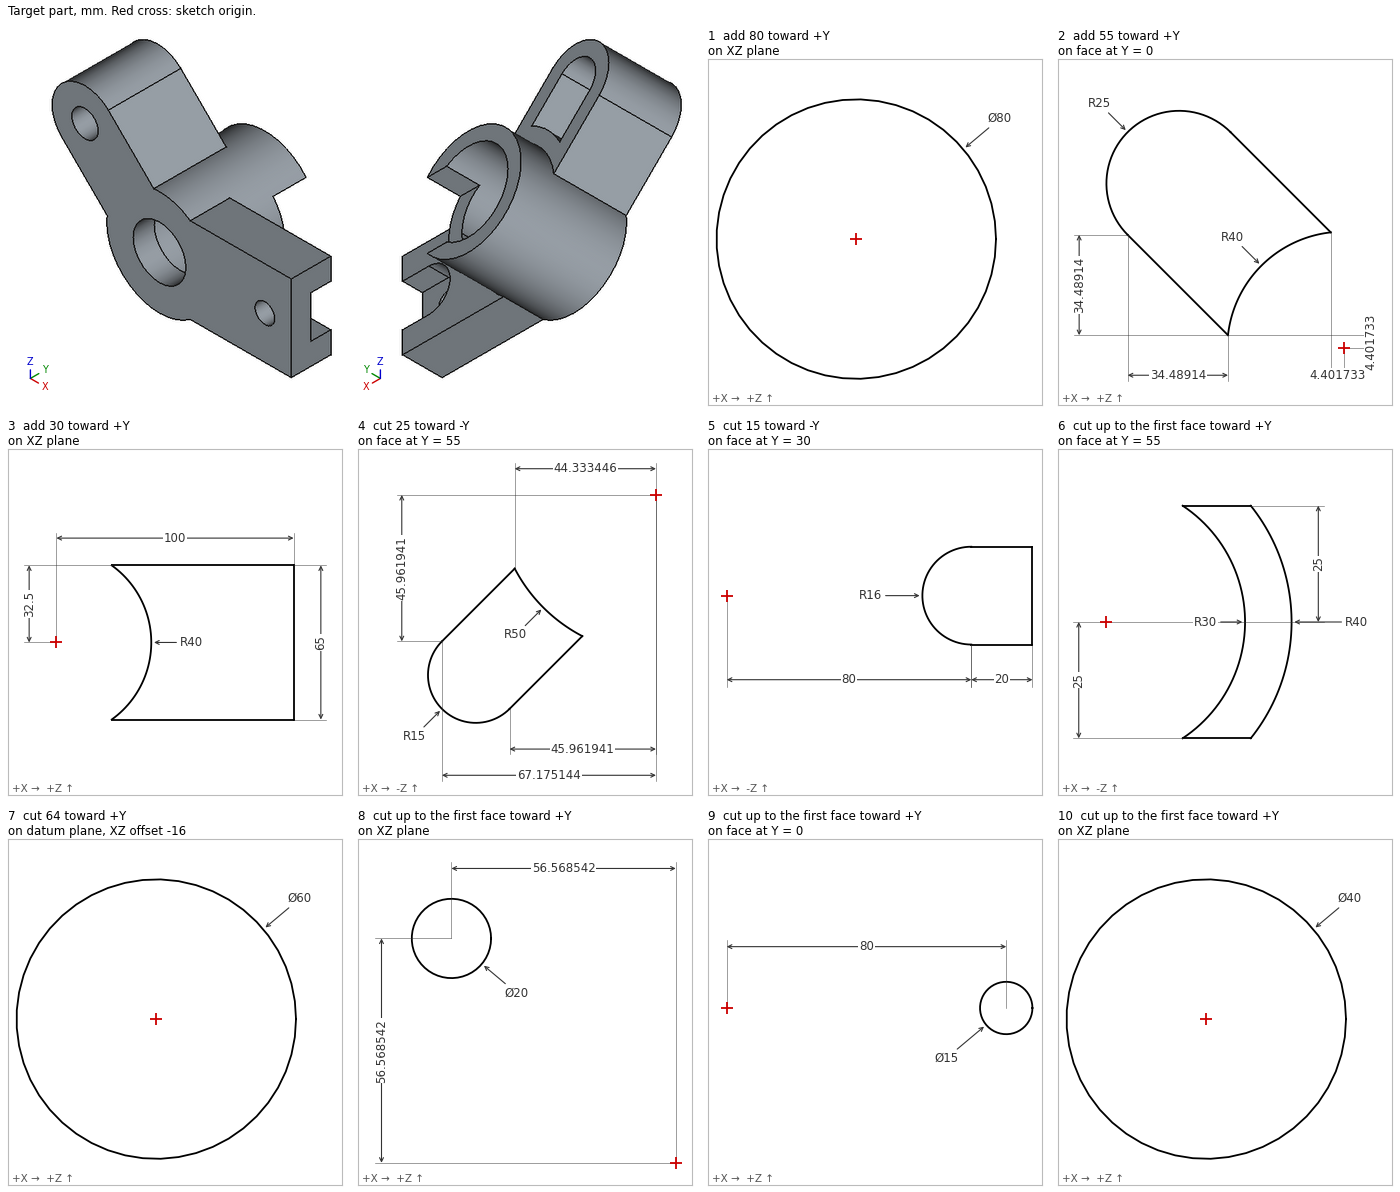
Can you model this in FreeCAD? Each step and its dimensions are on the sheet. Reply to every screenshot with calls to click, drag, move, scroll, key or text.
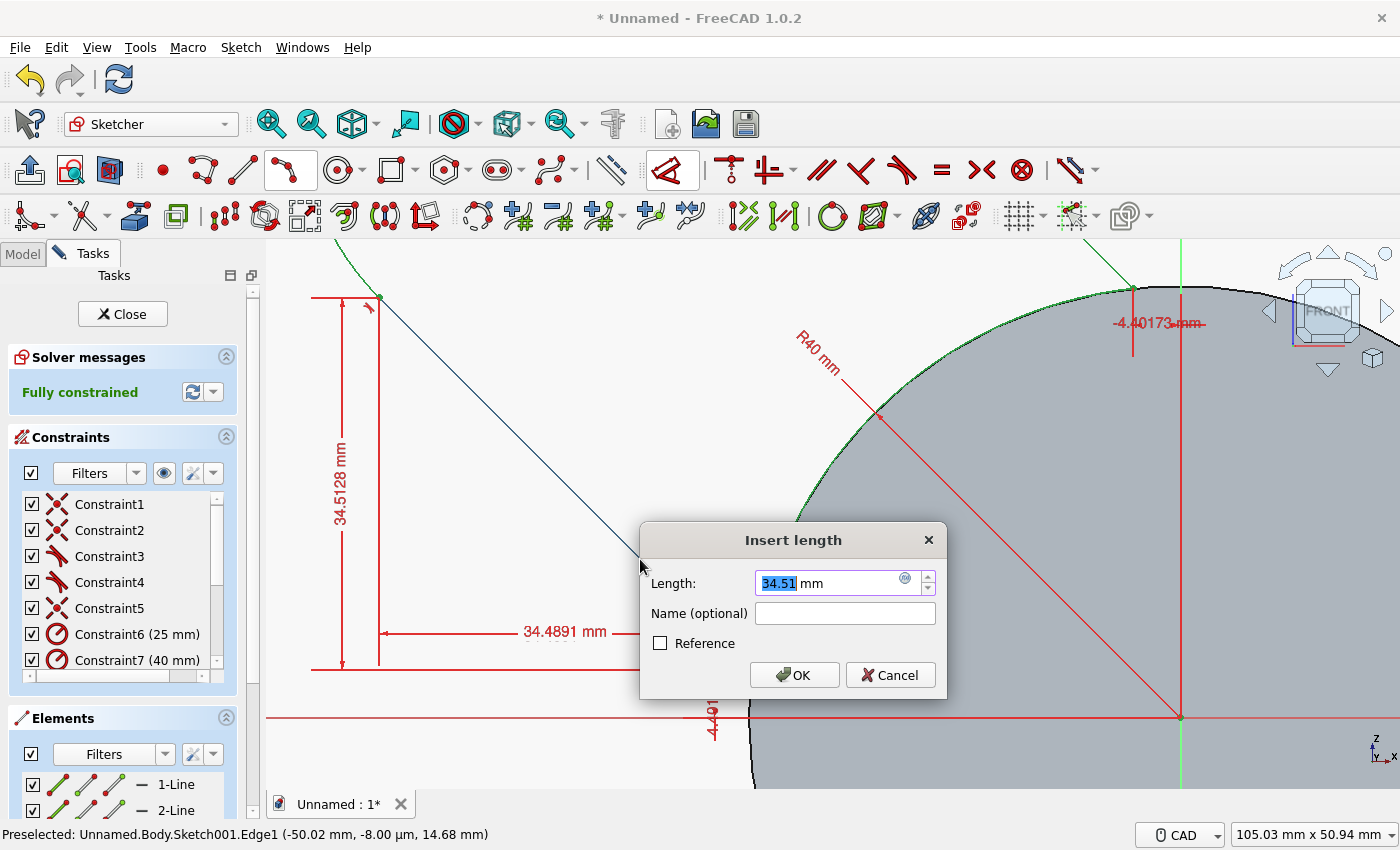
text(34.48914)
key(Return)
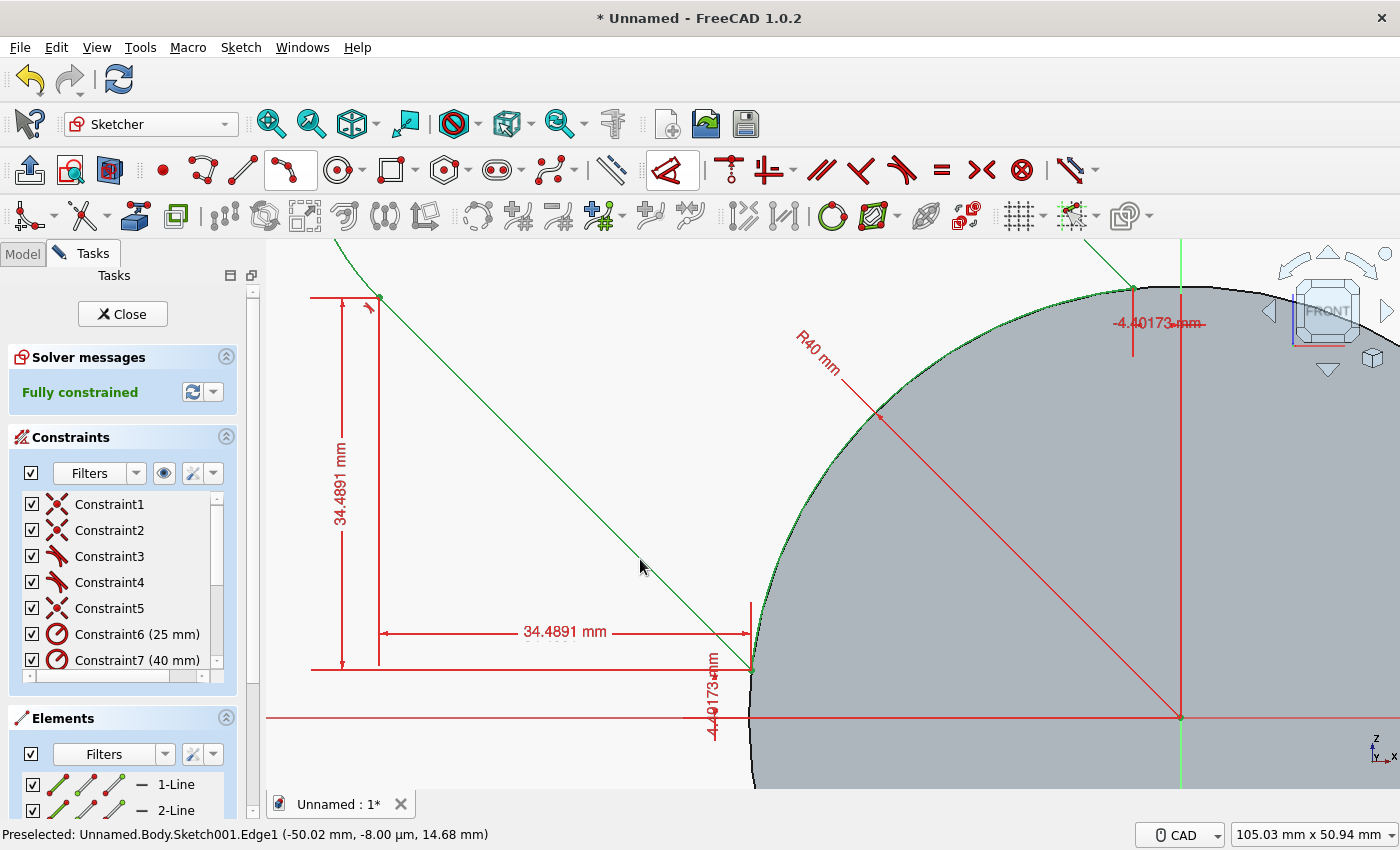
click(123, 314)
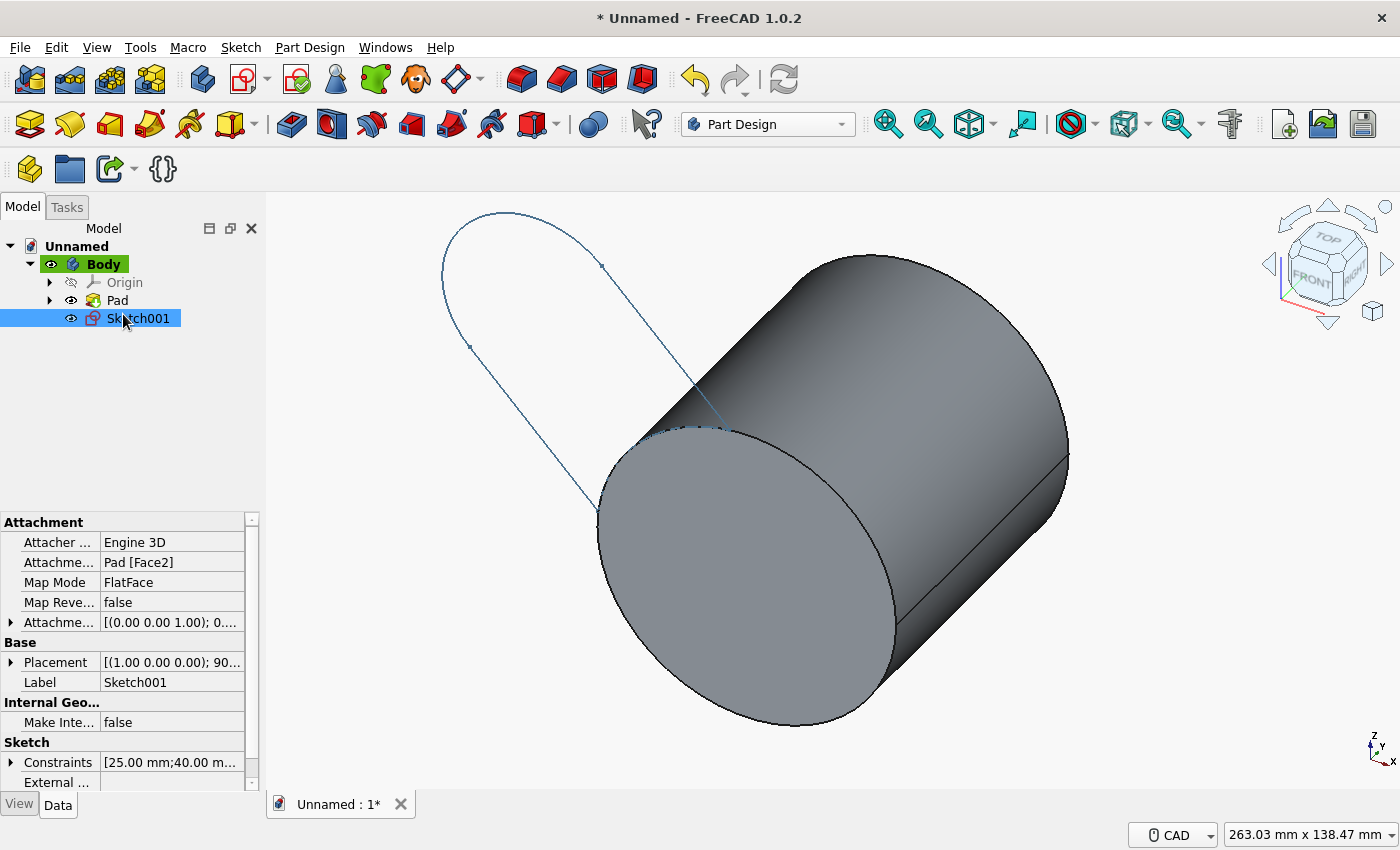
click(30, 124)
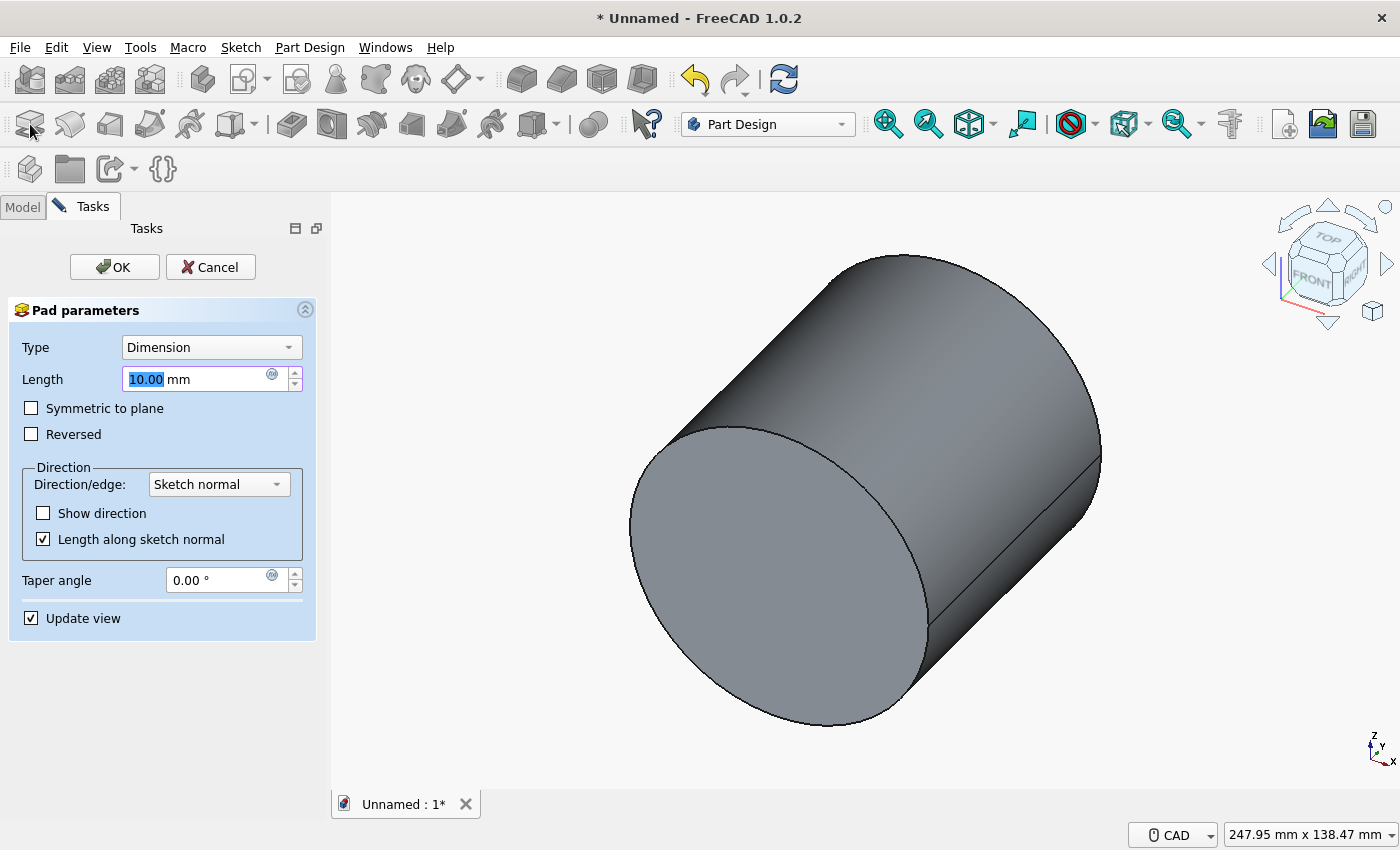
text(55)
key(Tab)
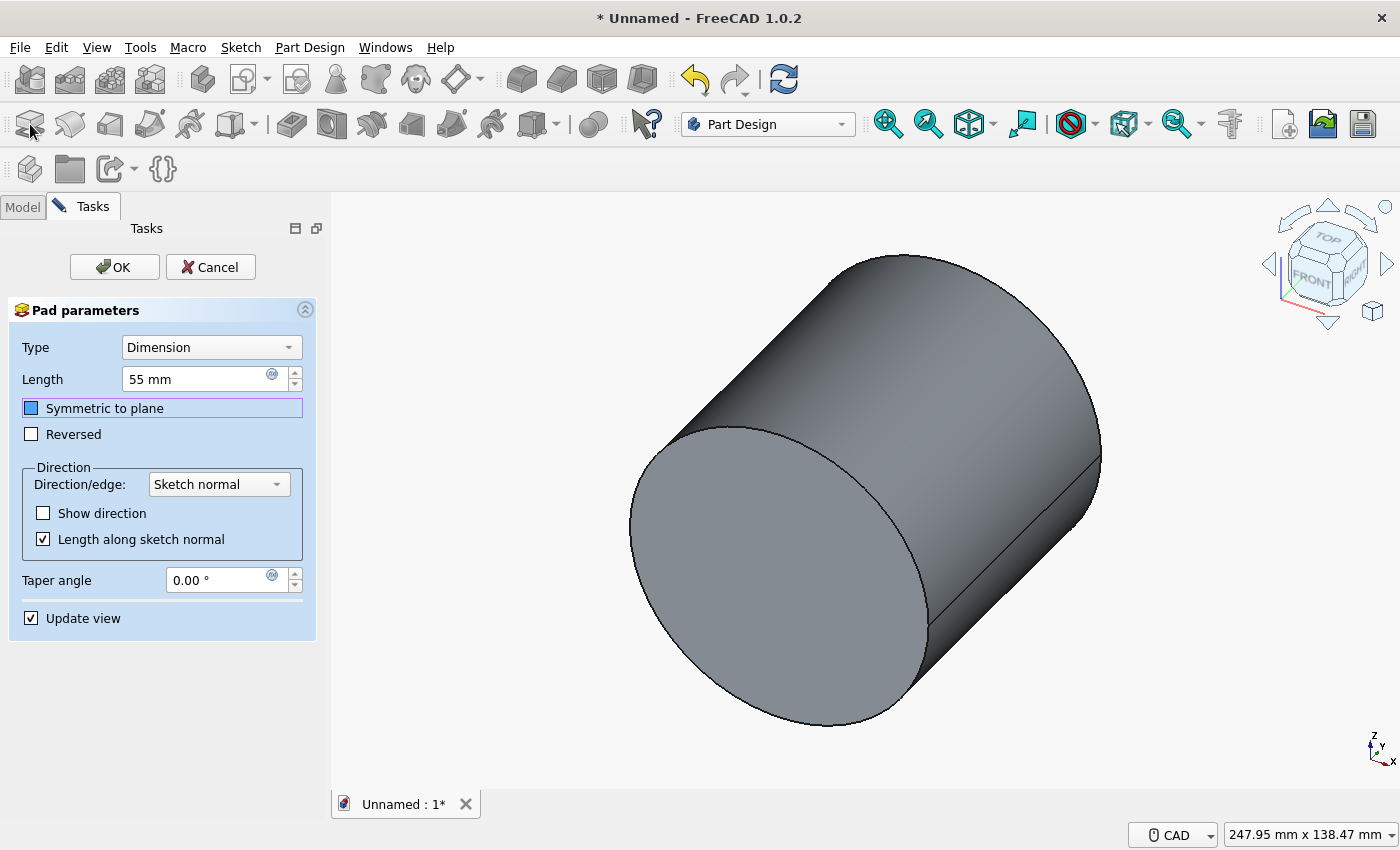
click(30, 434)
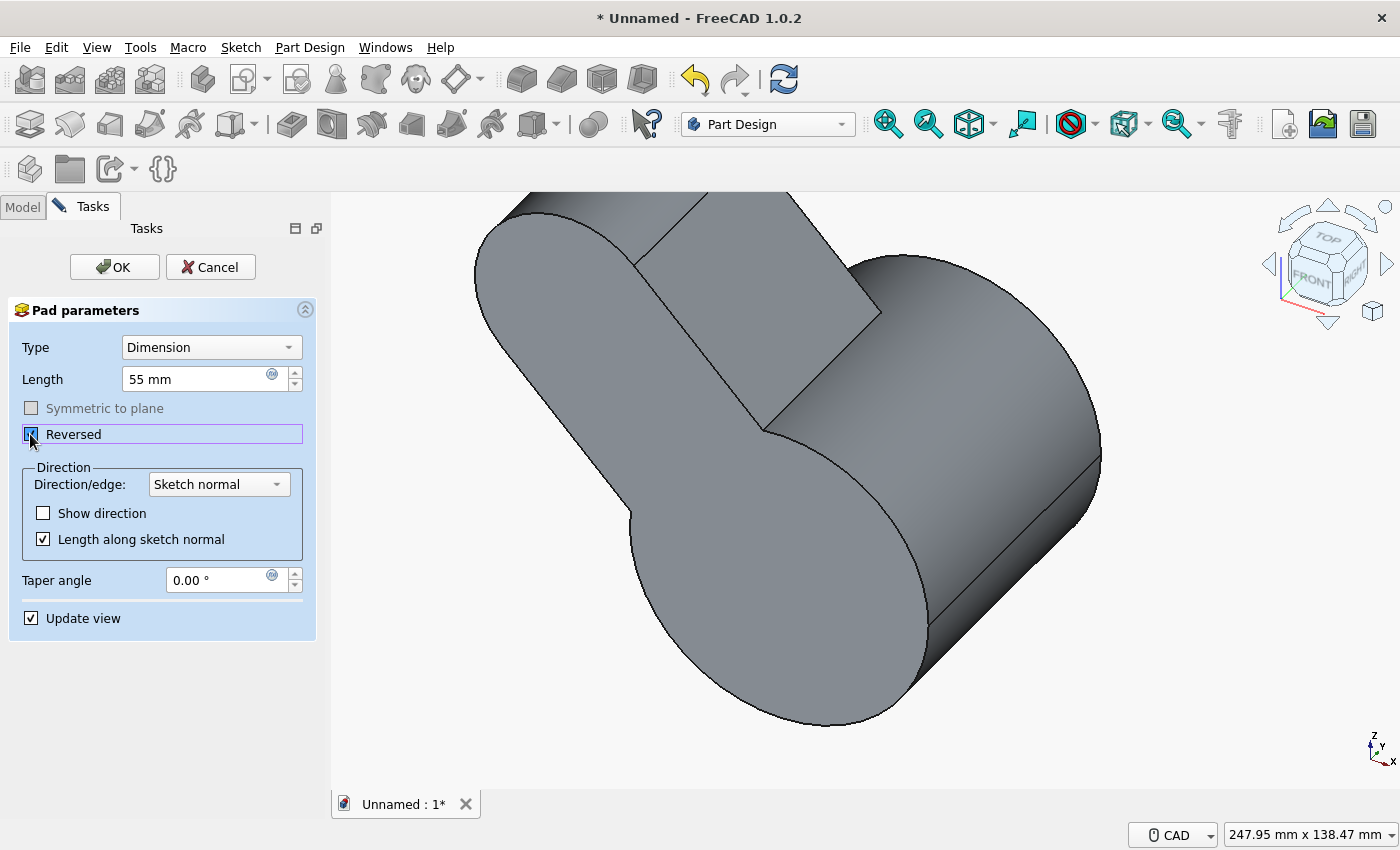
click(115, 267)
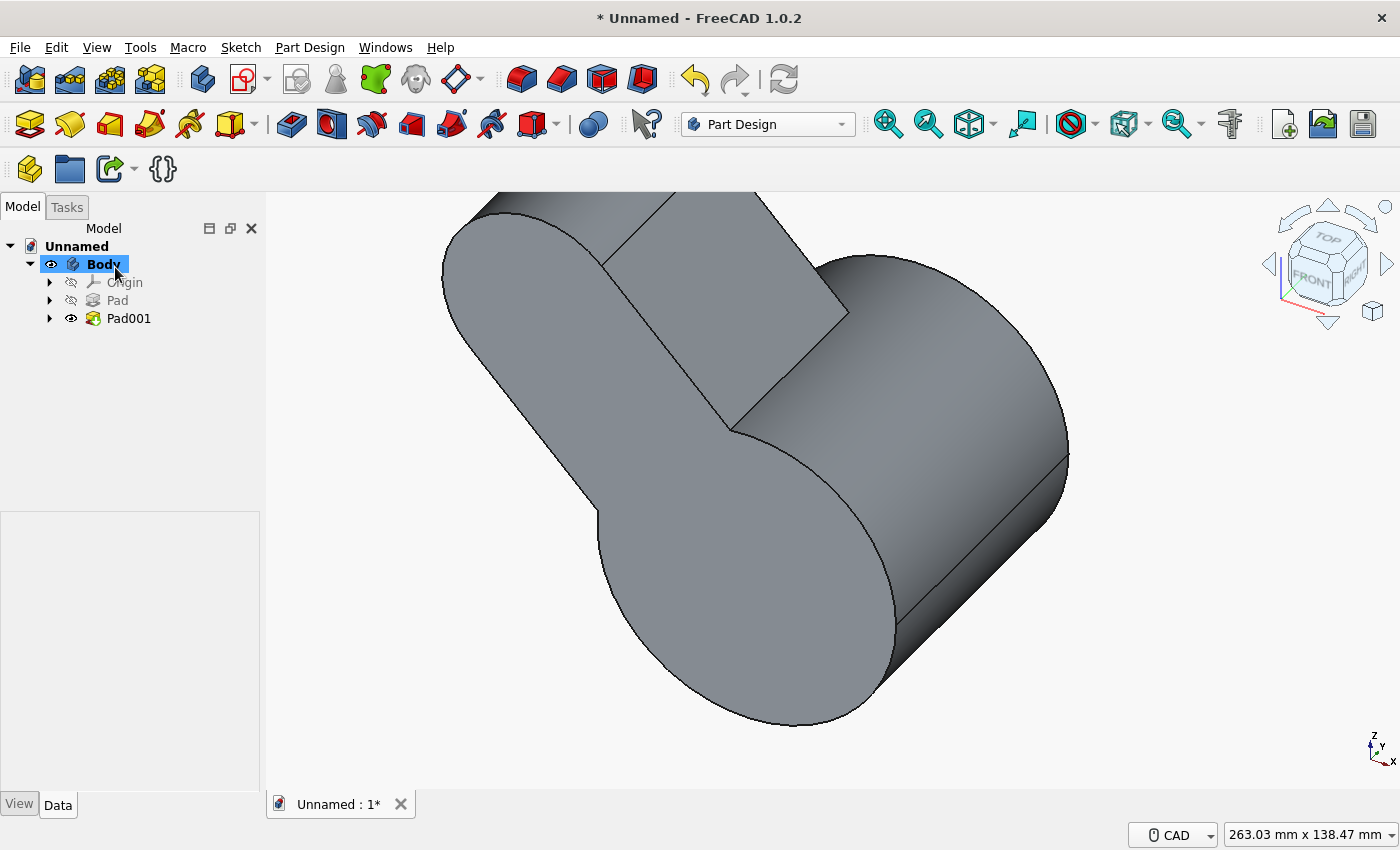
key(v)
key(f)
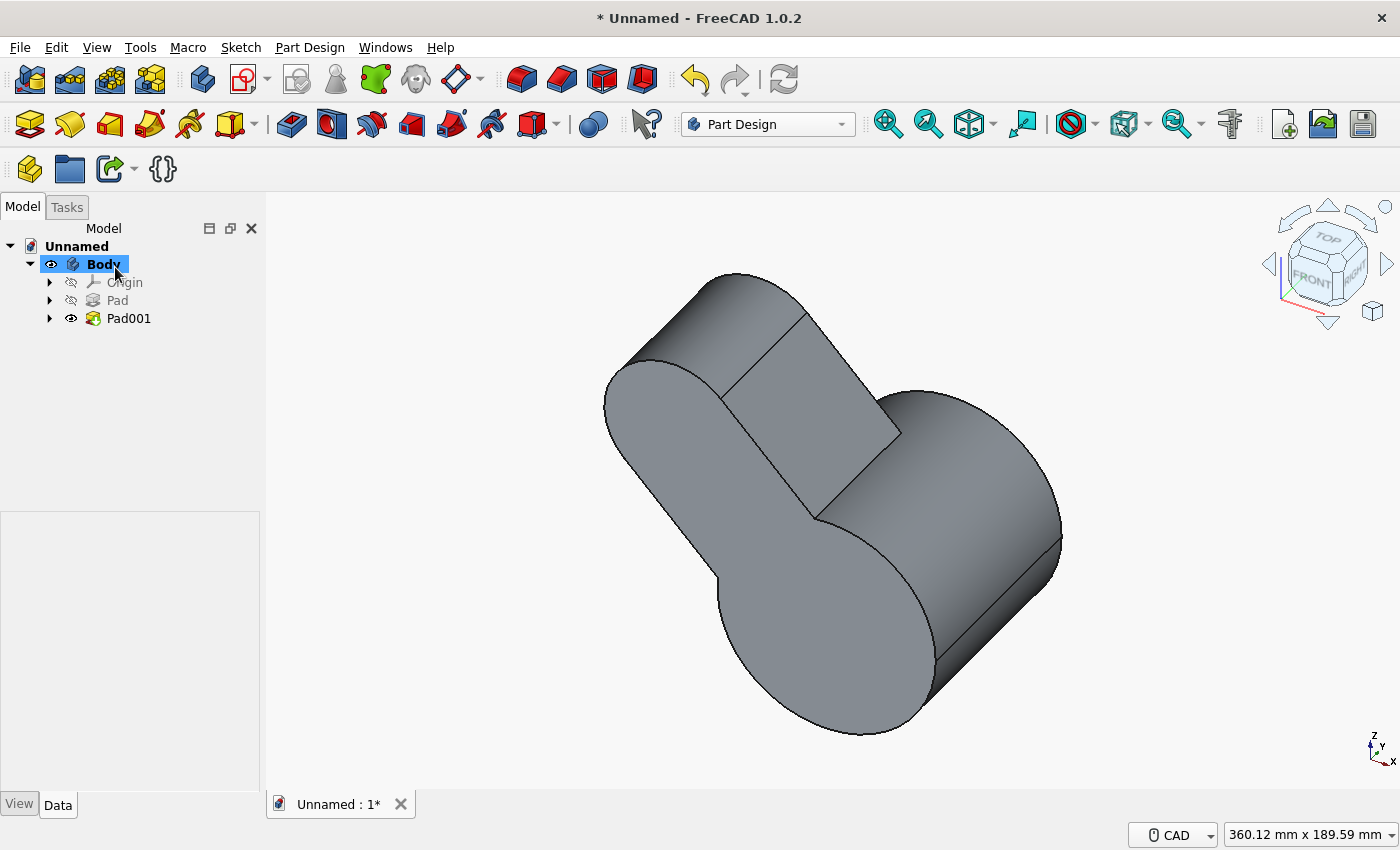
click(244, 80)